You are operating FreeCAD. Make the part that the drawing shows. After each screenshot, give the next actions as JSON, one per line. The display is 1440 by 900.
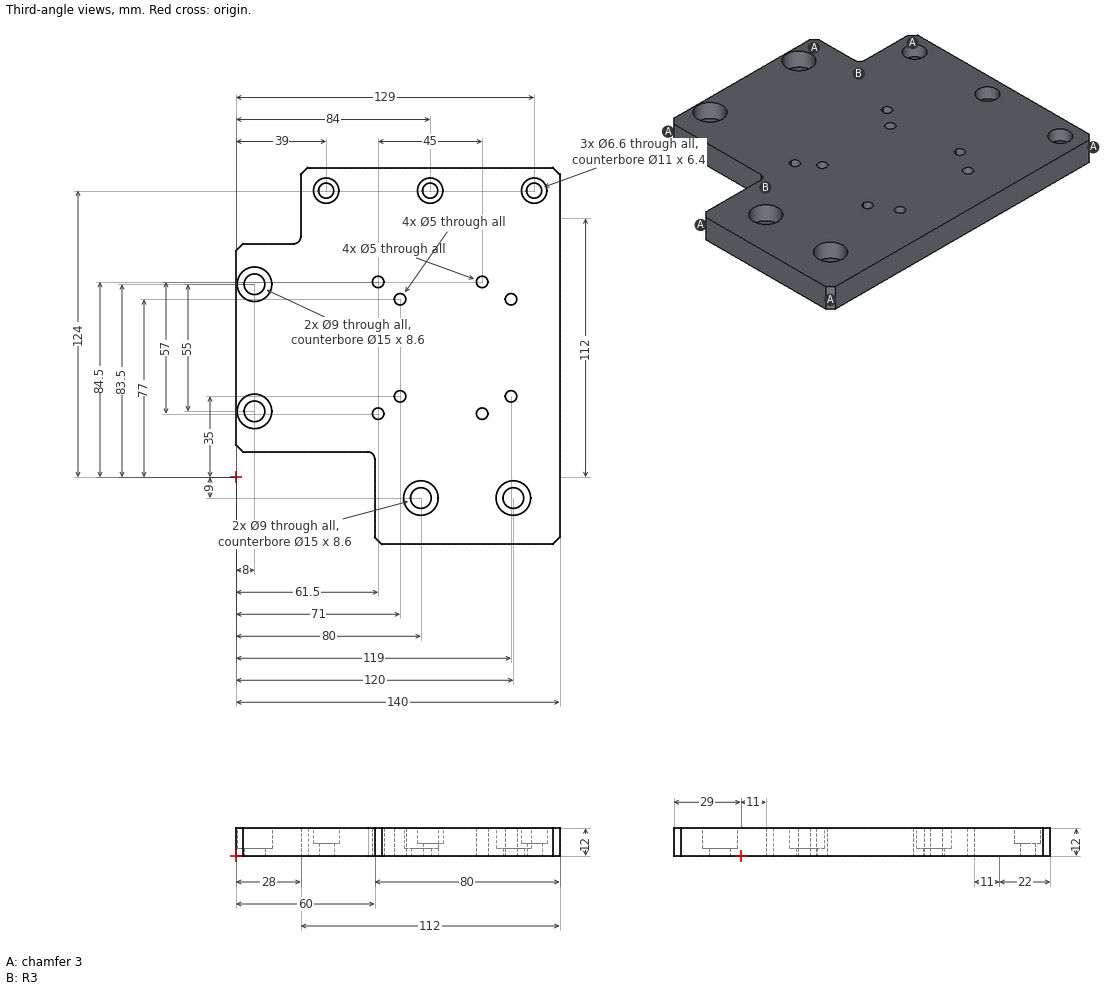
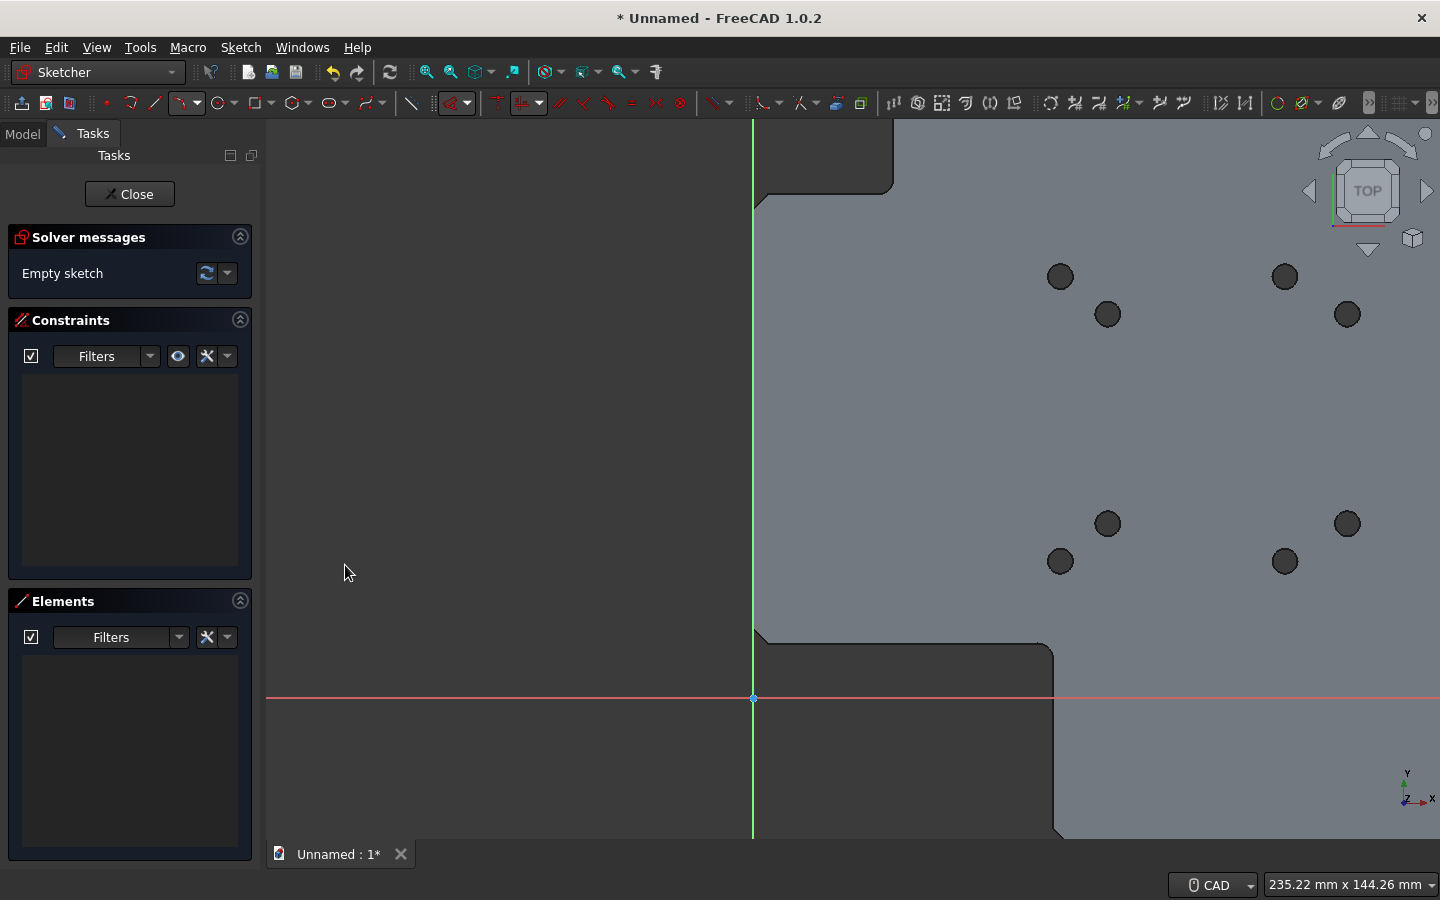
{"action": "key", "text": "g c"}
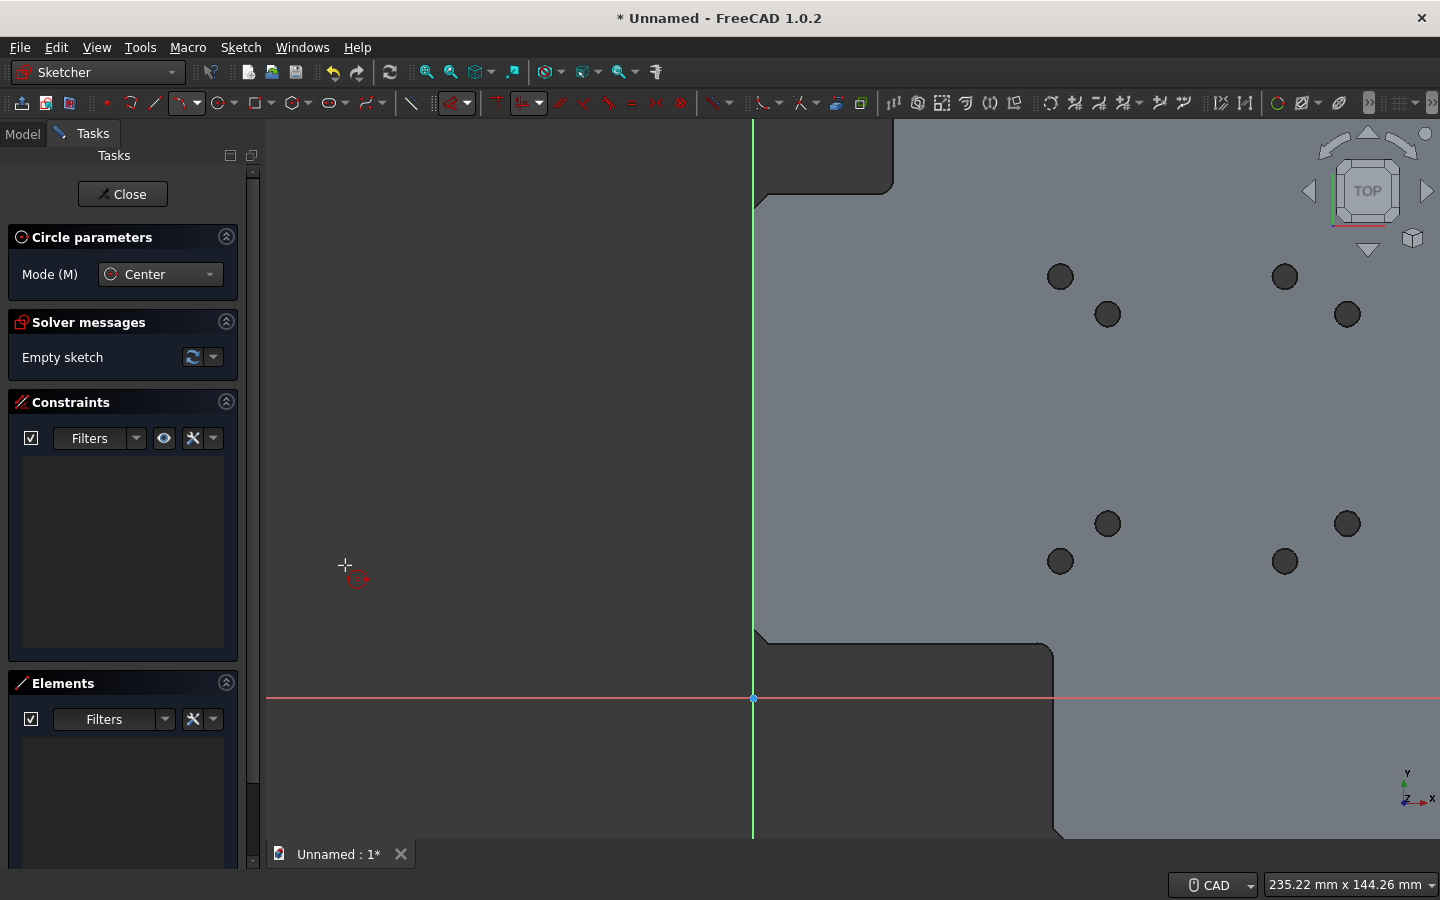
{"action": "left_click", "coordinate": [793, 282]}
{"action": "mouse_move", "coordinate": [809, 266]}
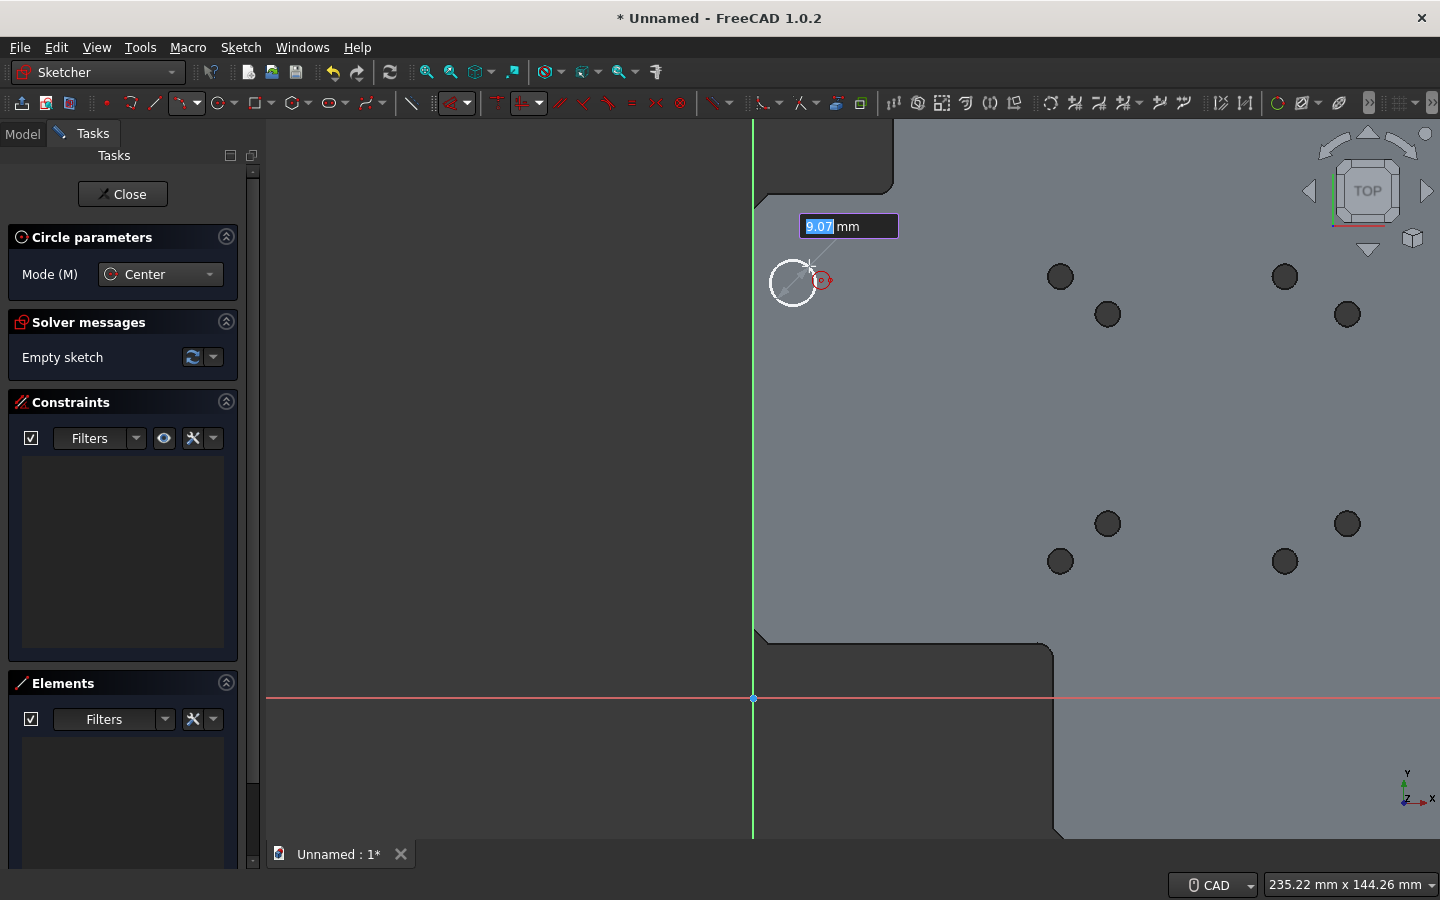
{"action": "type", "text": "9"}
{"action": "key", "text": "Return"}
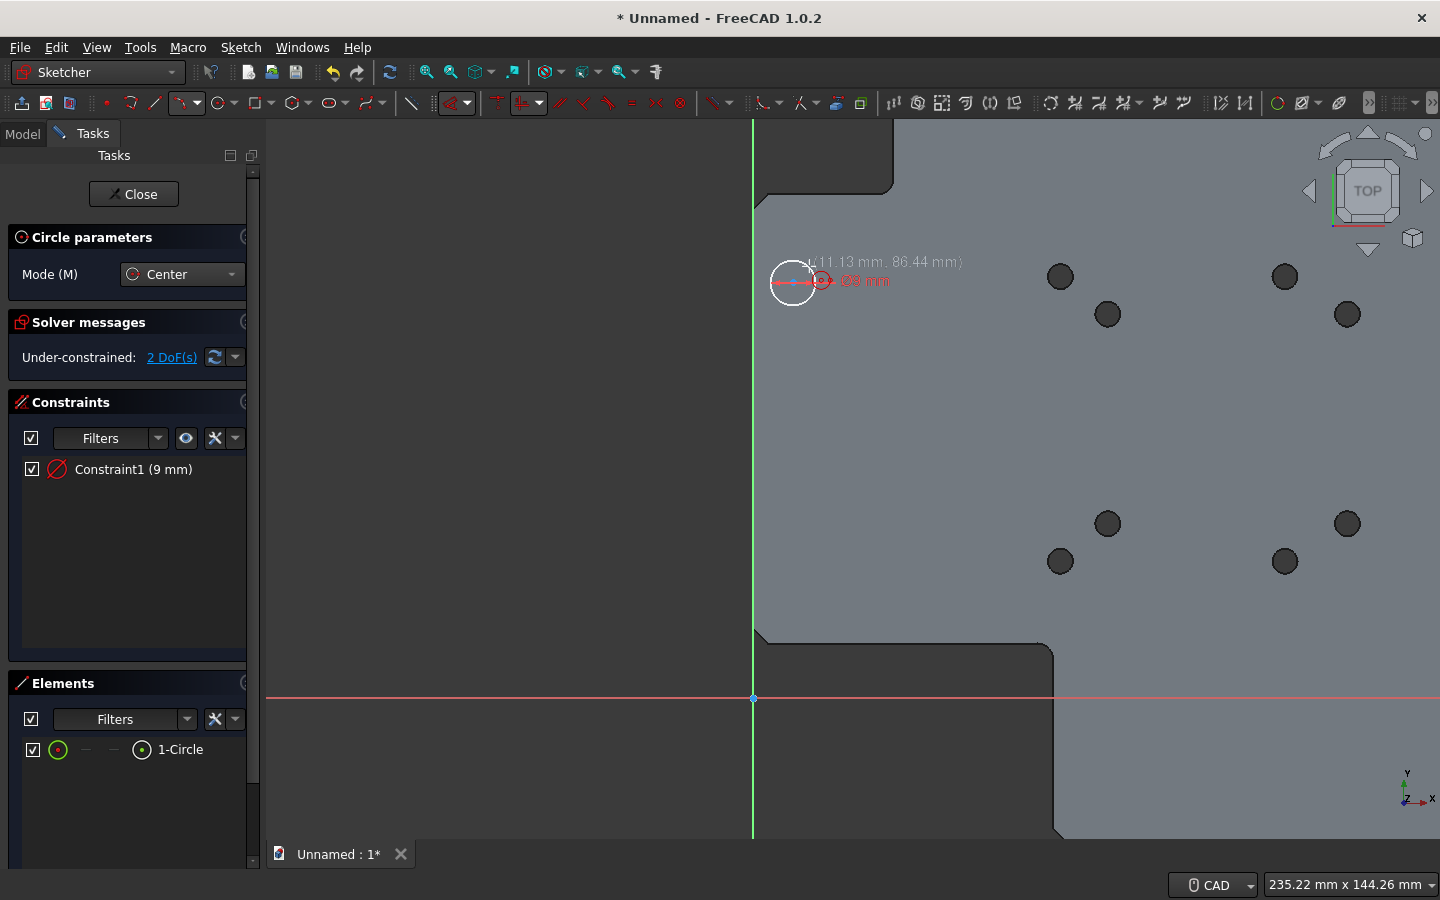
{"action": "left_click", "coordinate": [793, 556]}
{"action": "mouse_move", "coordinate": [809, 540]}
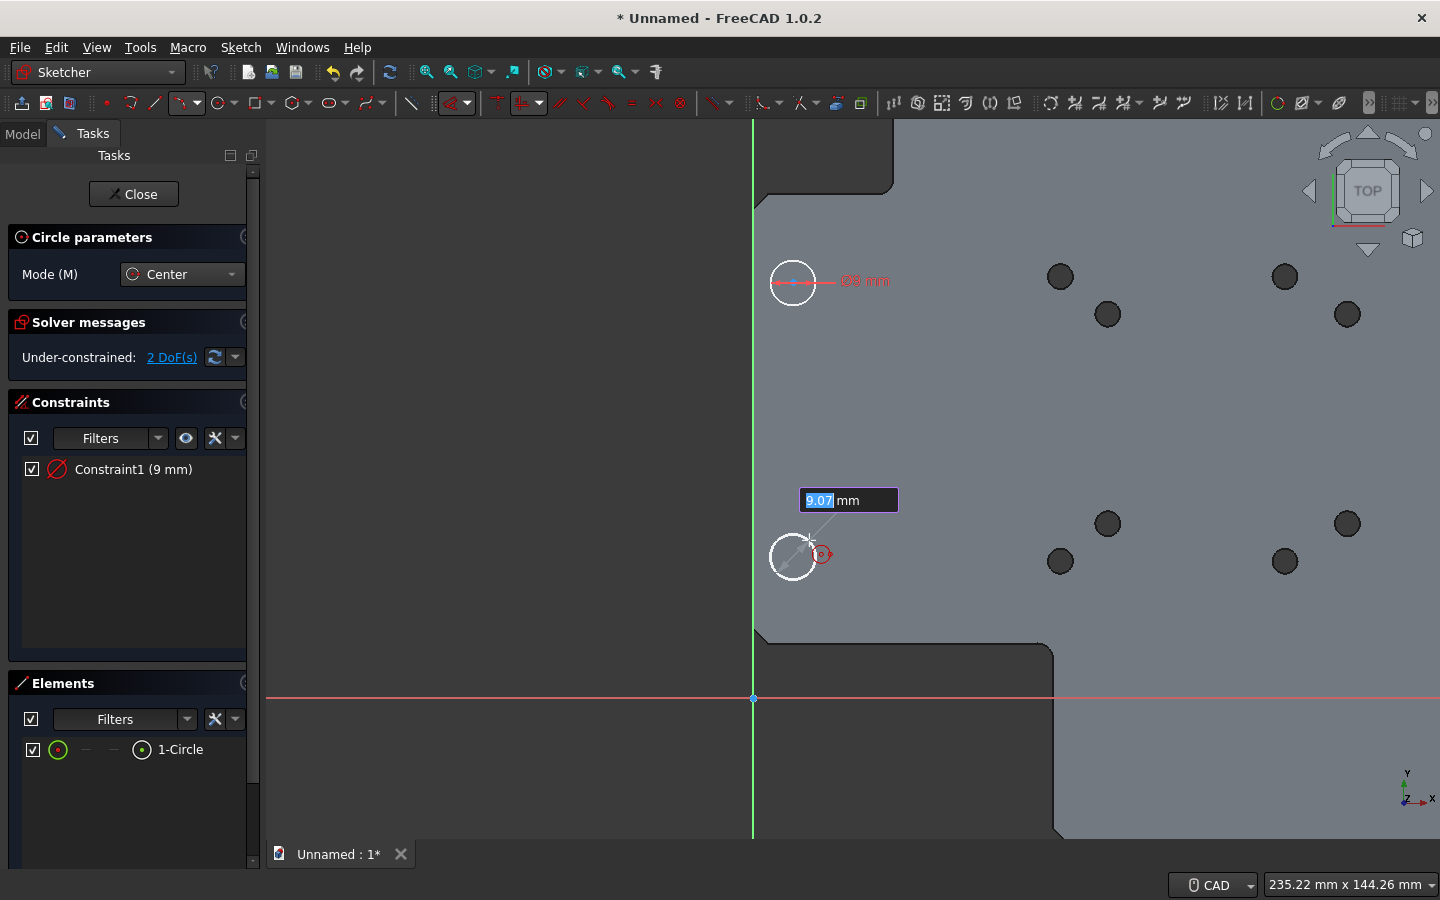
{"action": "type", "text": "9"}
{"action": "key", "text": "Return"}
{"action": "key", "text": "Escape"}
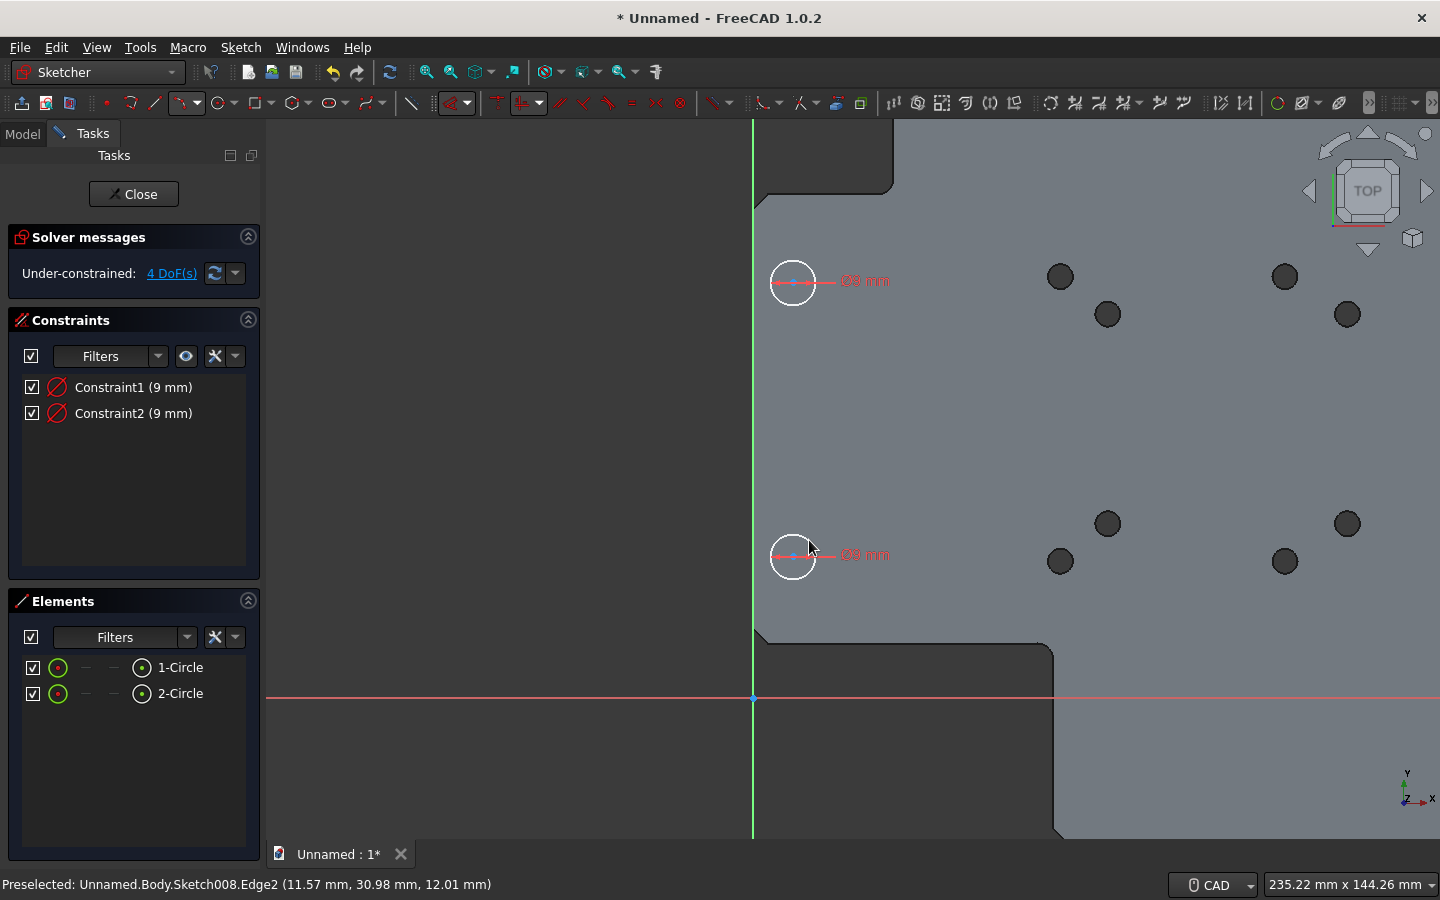
{"action": "left_click", "coordinate": [793, 283]}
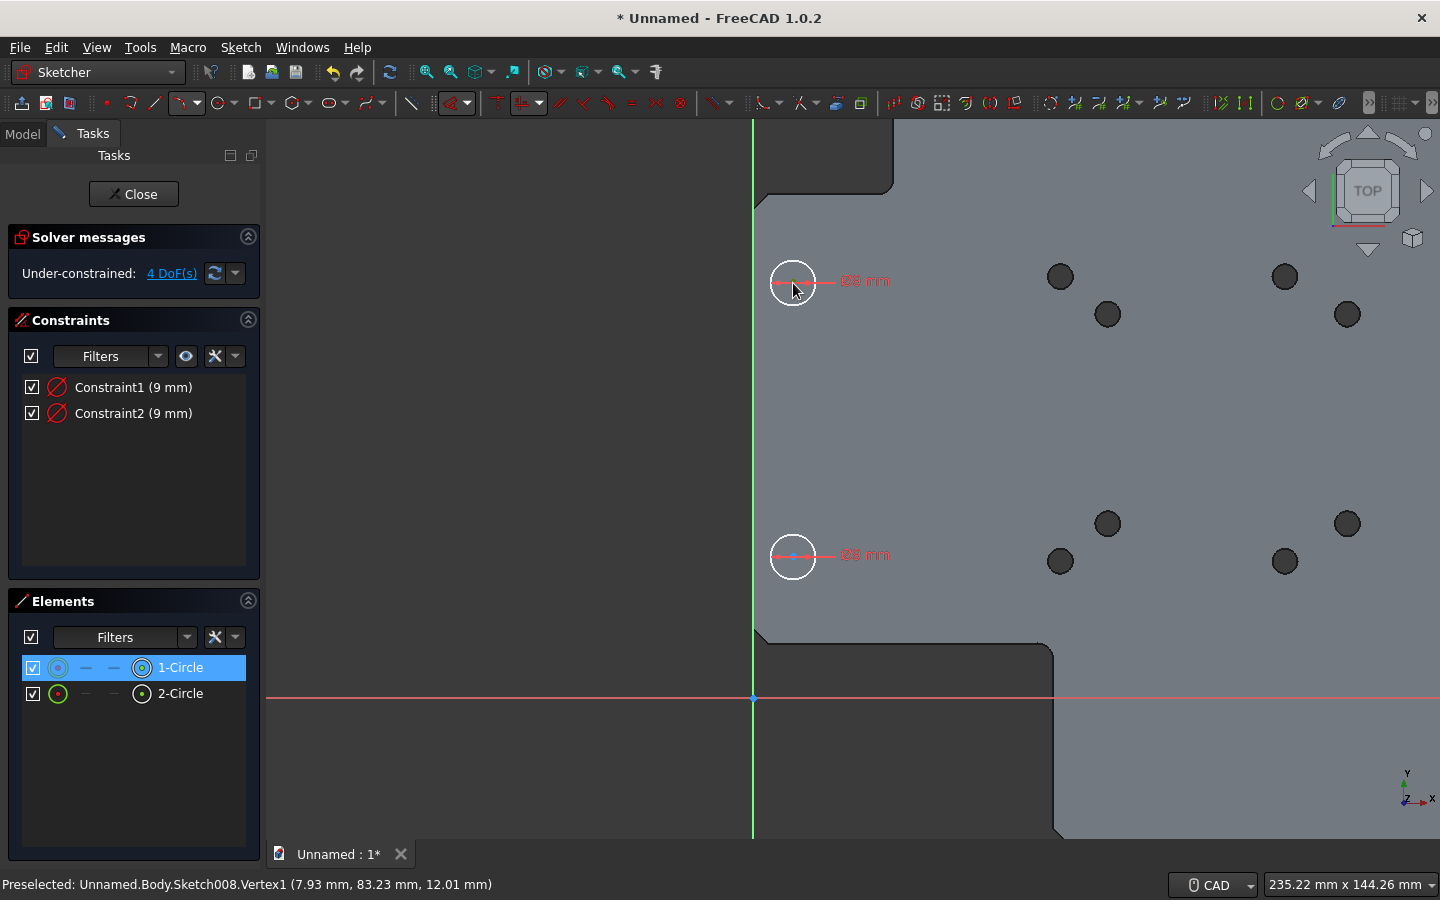
{"action": "key", "text": "l"}